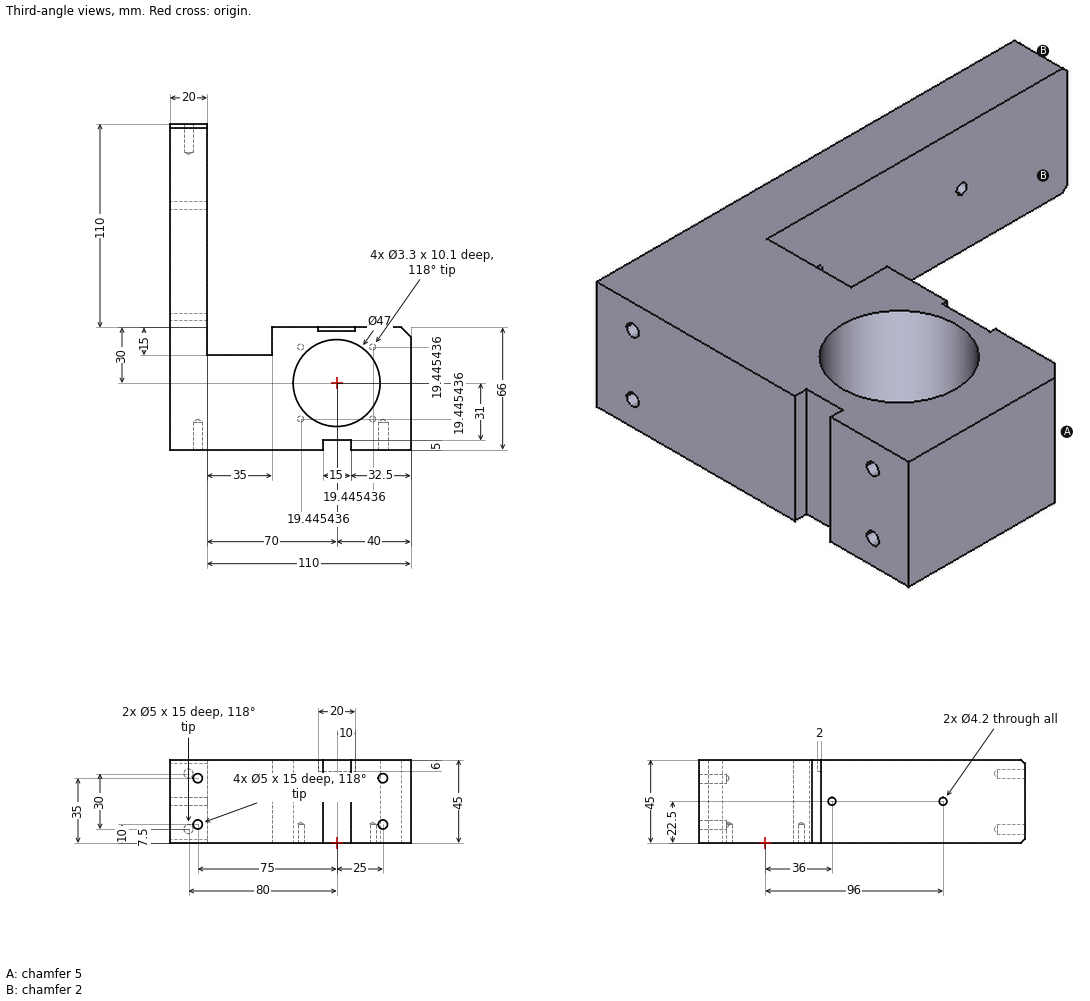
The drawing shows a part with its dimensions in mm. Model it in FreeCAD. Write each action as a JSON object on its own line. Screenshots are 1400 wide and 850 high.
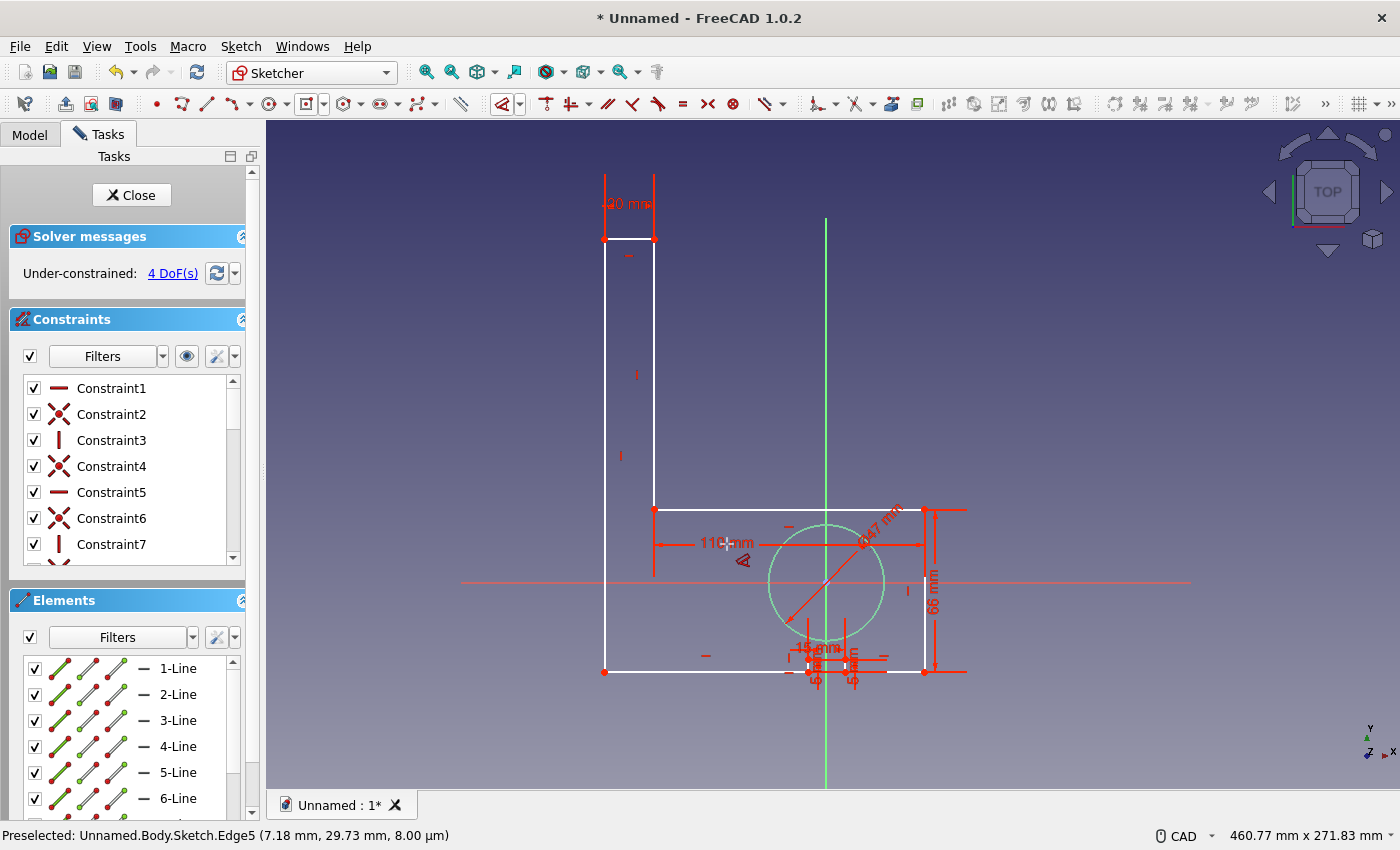
{"action": "left_click", "coordinate": [654, 429]}
{"action": "left_click", "coordinate": [620, 374]}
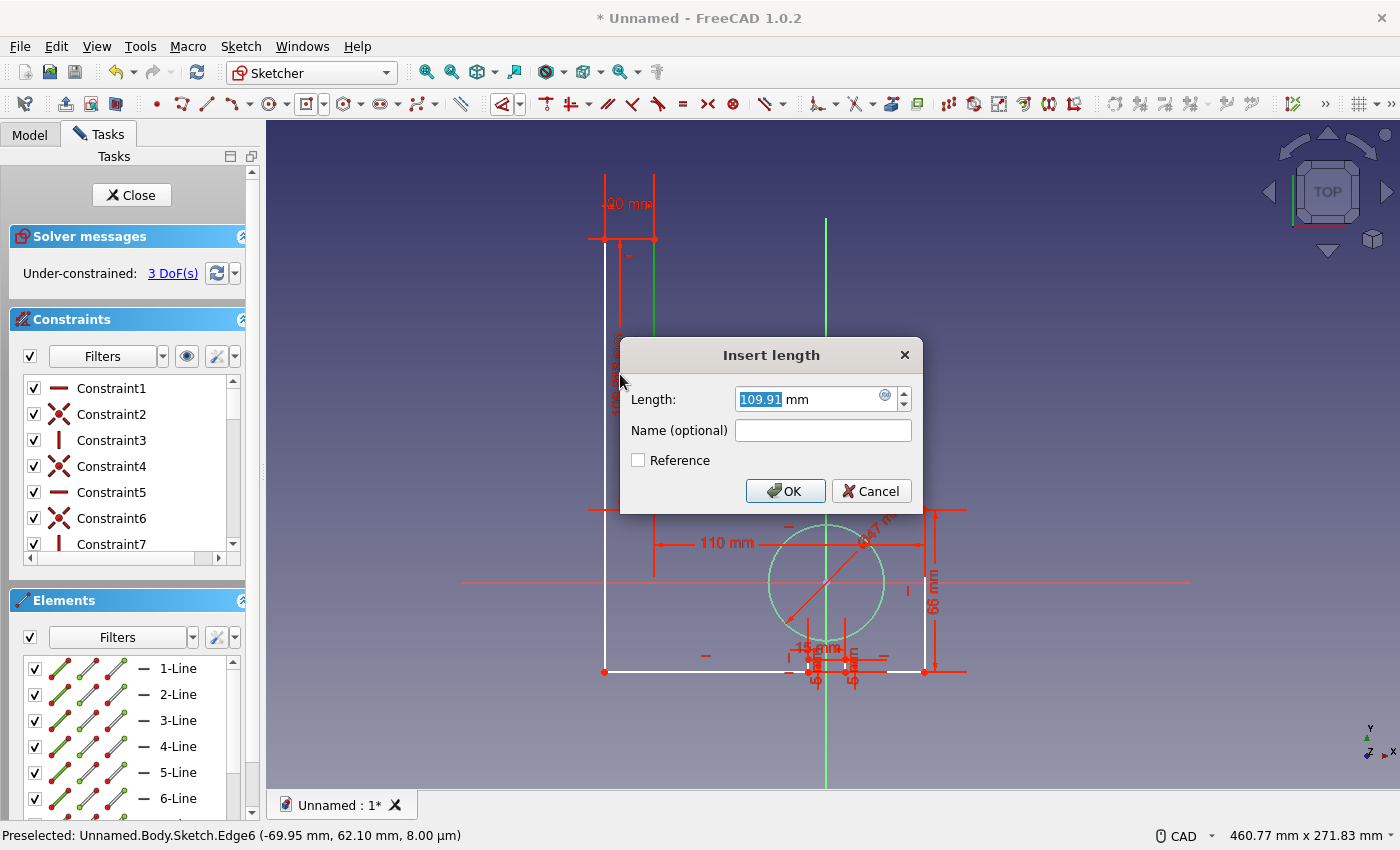
{"action": "type", "text": "110"}
{"action": "key", "text": "Return"}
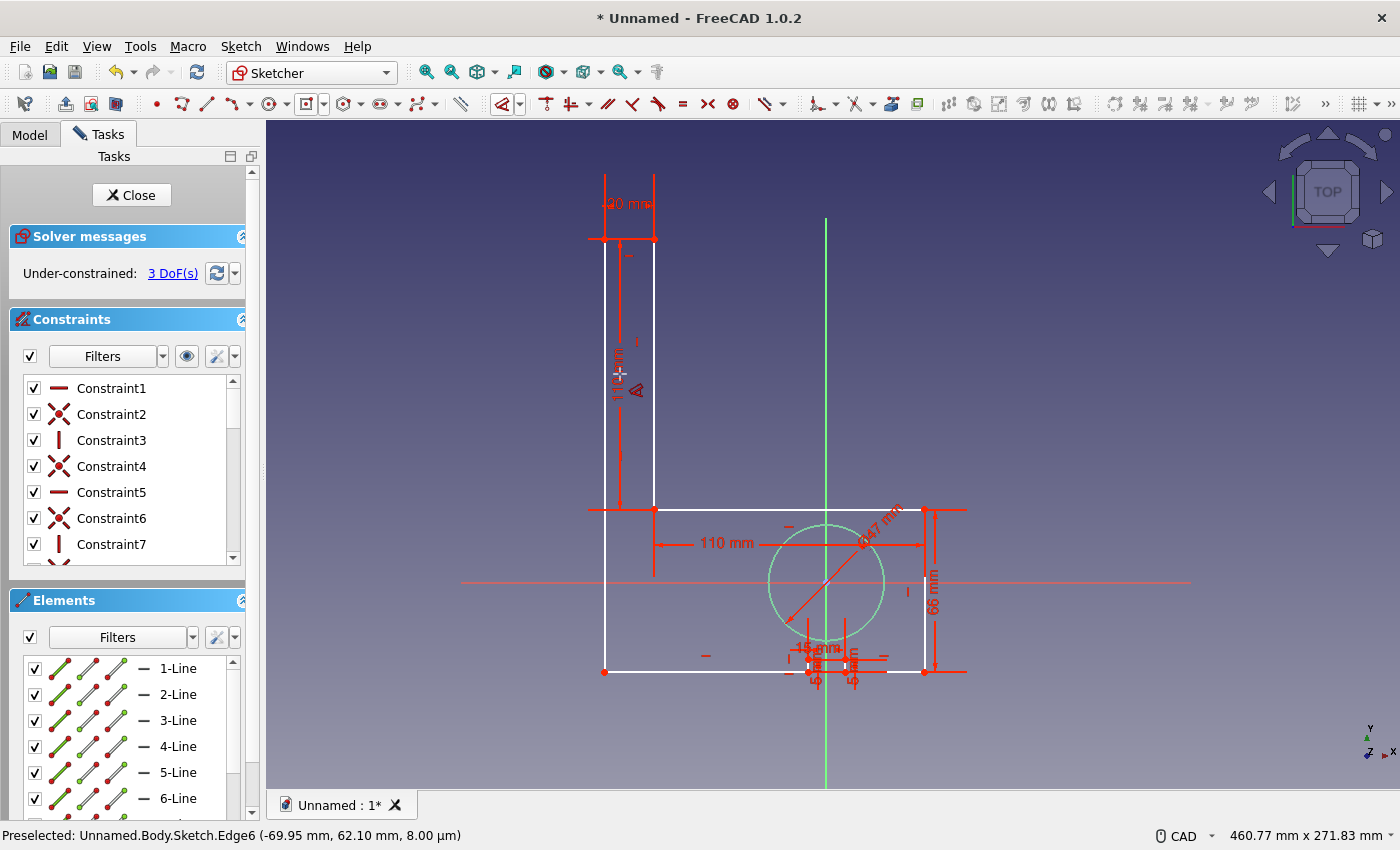
{"action": "left_click", "coordinate": [808, 660]}
{"action": "left_click", "coordinate": [860, 604]}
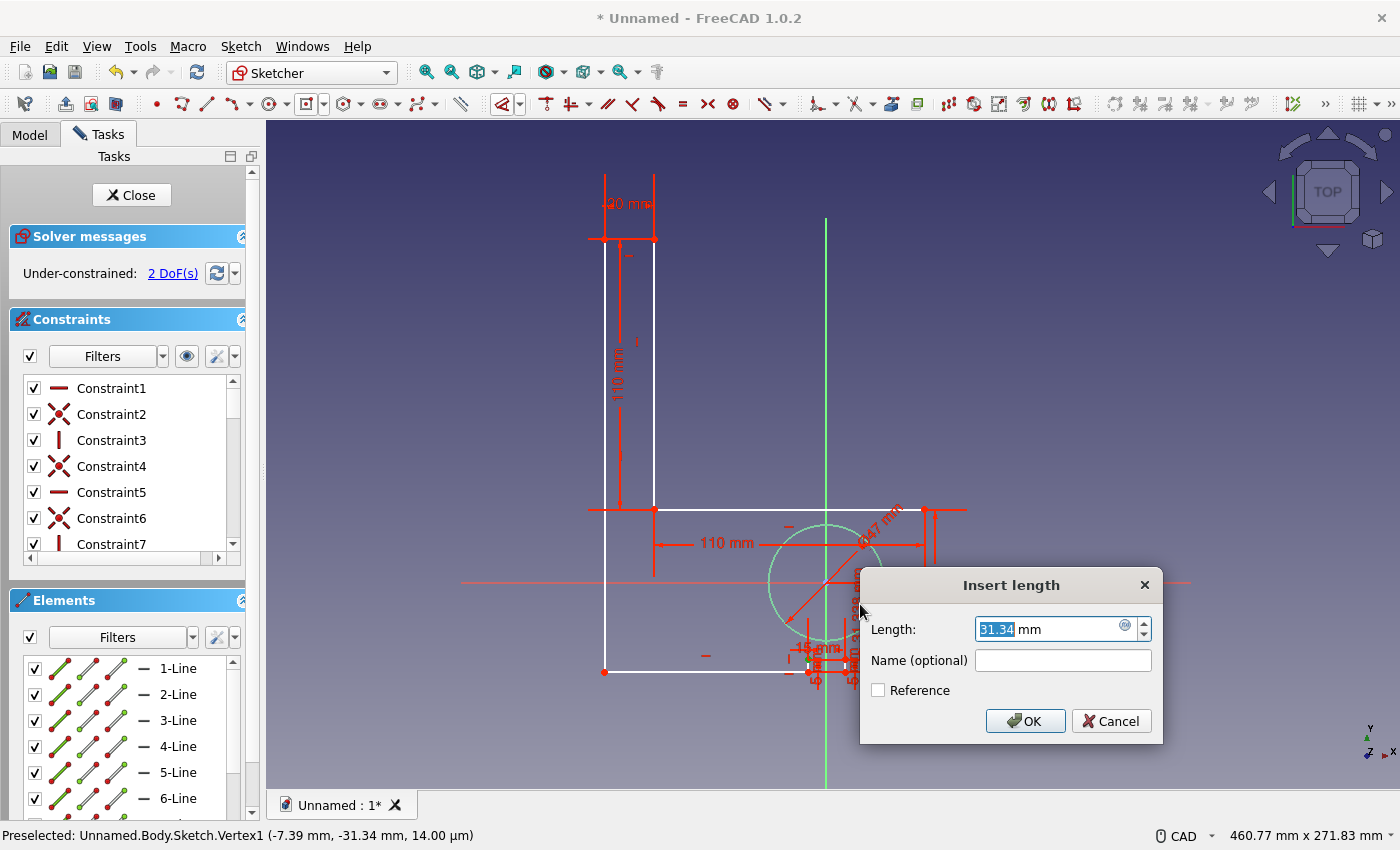
{"action": "type", "text": "31"}
{"action": "key", "text": "Return"}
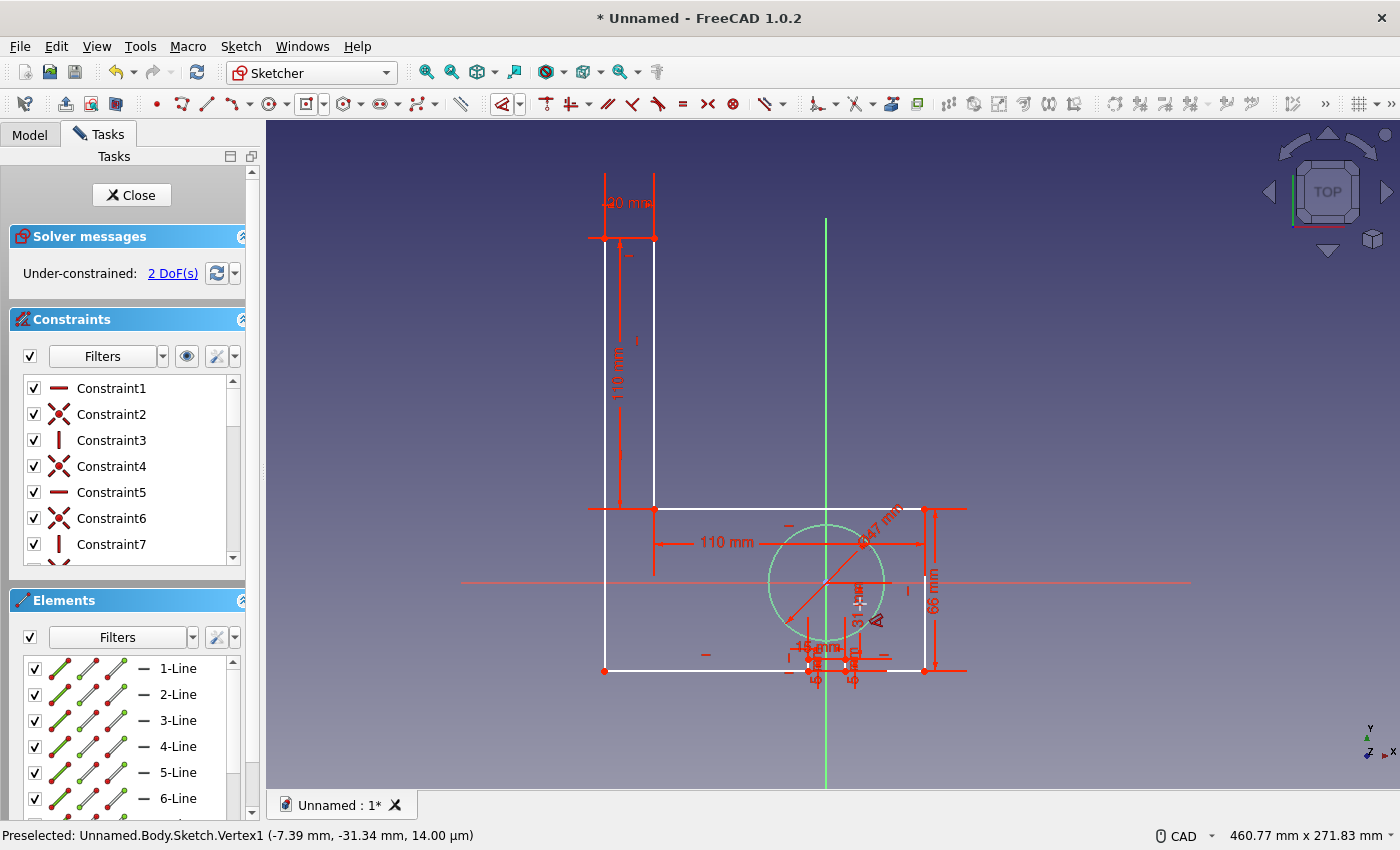
{"action": "left_click", "coordinate": [925, 671]}
{"action": "left_click", "coordinate": [876, 705]}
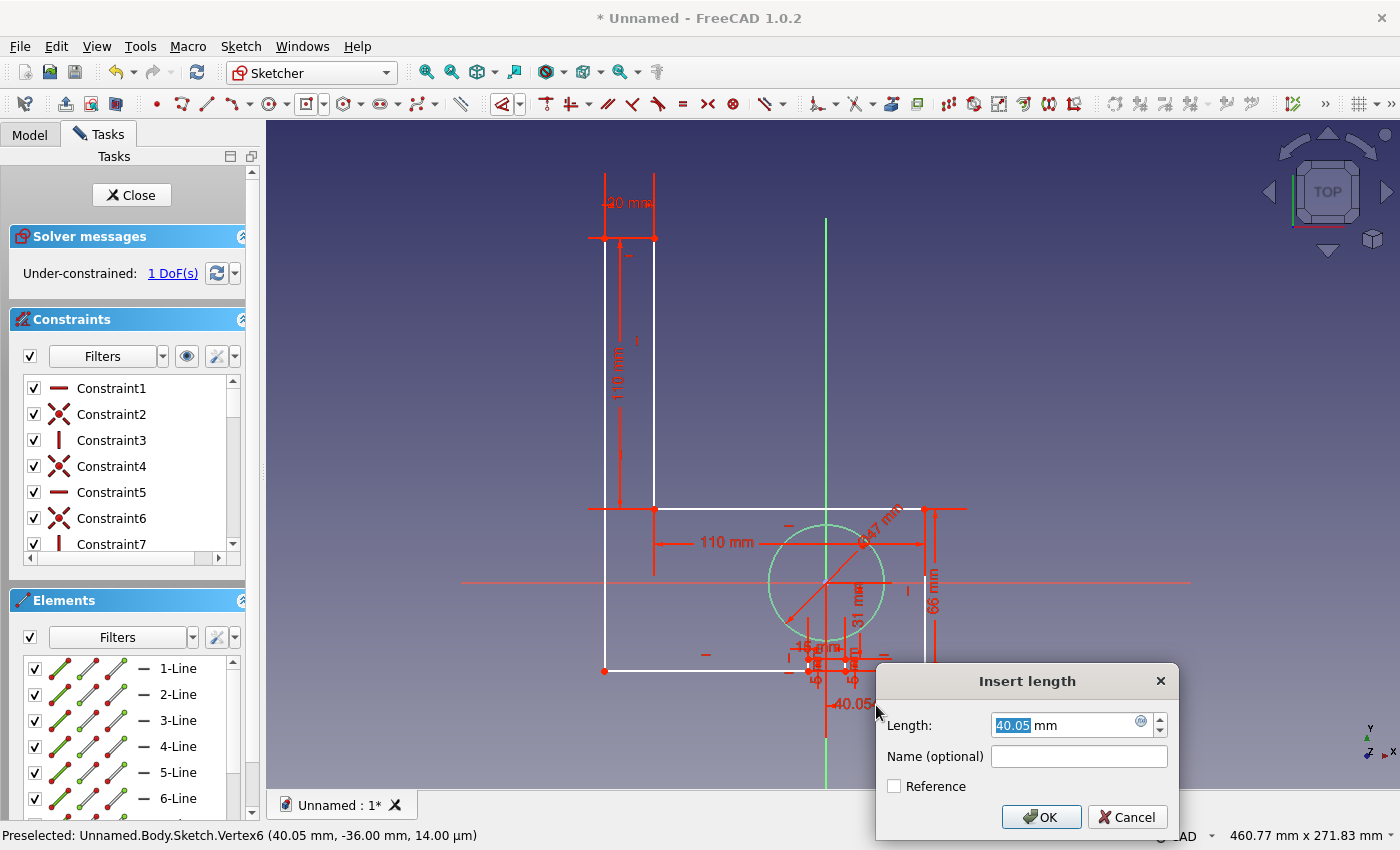
{"action": "type", "text": "40"}
{"action": "key", "text": "Return"}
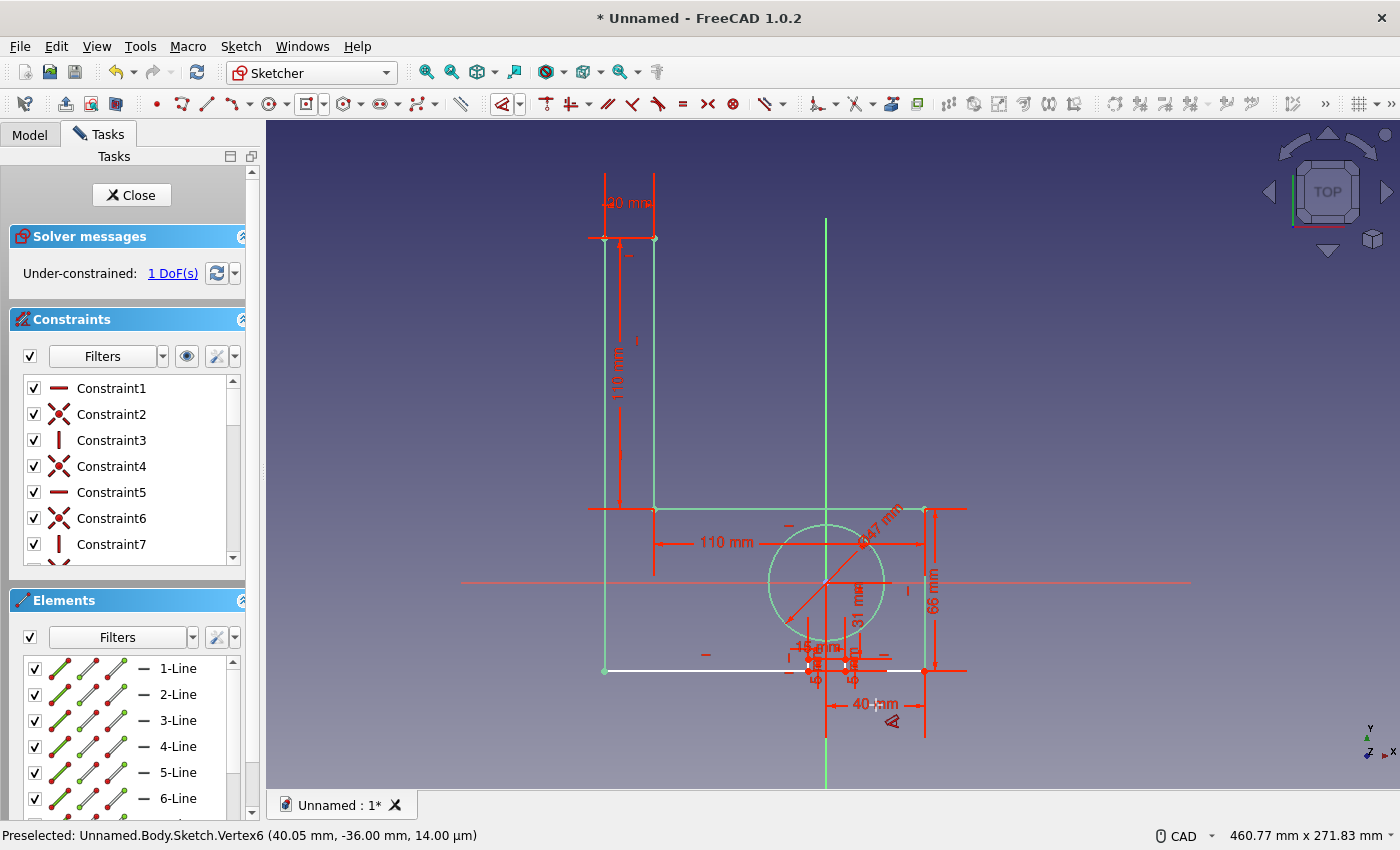
{"action": "left_click", "coordinate": [869, 671]}
{"action": "left_click", "coordinate": [903, 637]}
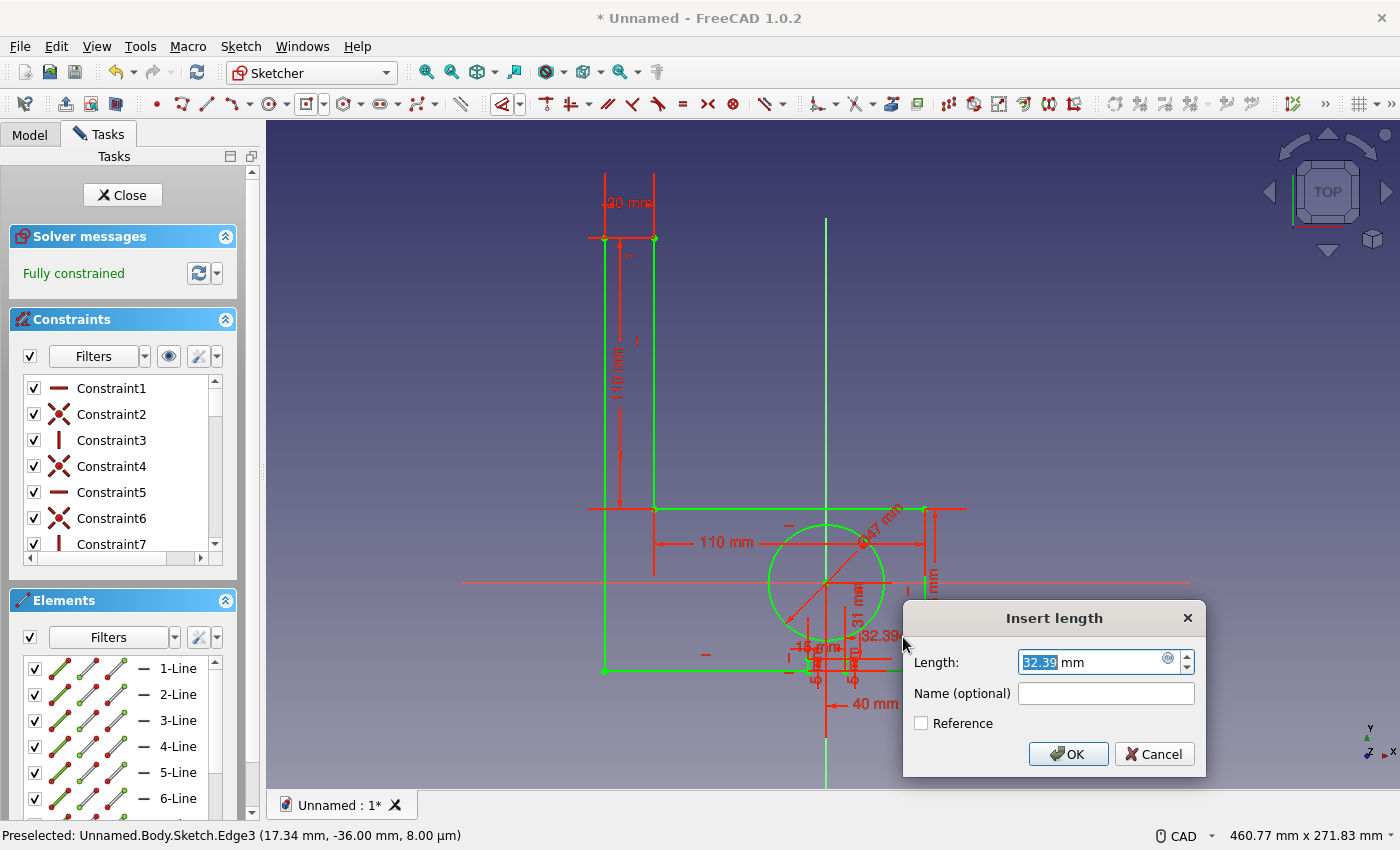
{"action": "type", "text": "32.5"}
{"action": "key", "text": "Return"}
{"action": "key", "text": "Escape"}